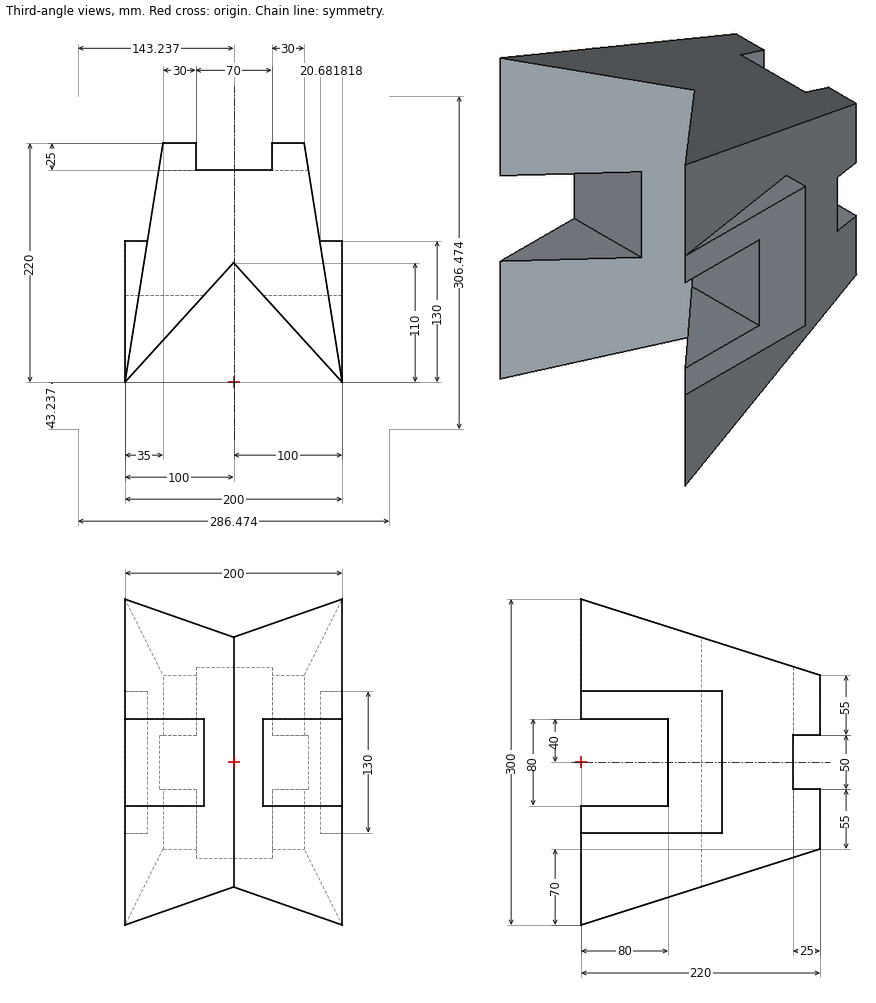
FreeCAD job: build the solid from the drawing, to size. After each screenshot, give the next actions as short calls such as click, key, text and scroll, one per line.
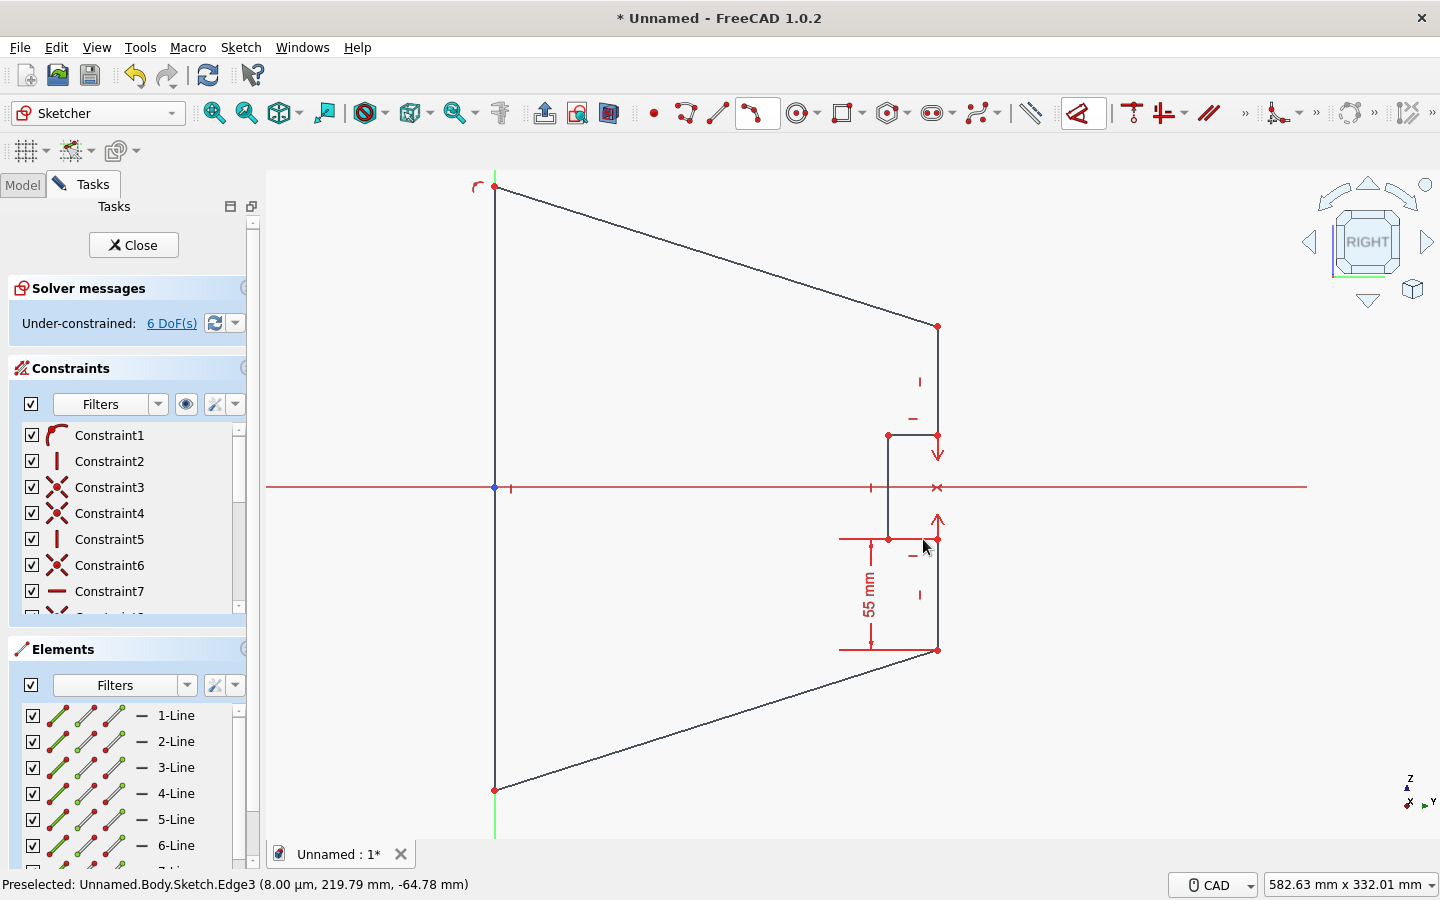
click(923, 539)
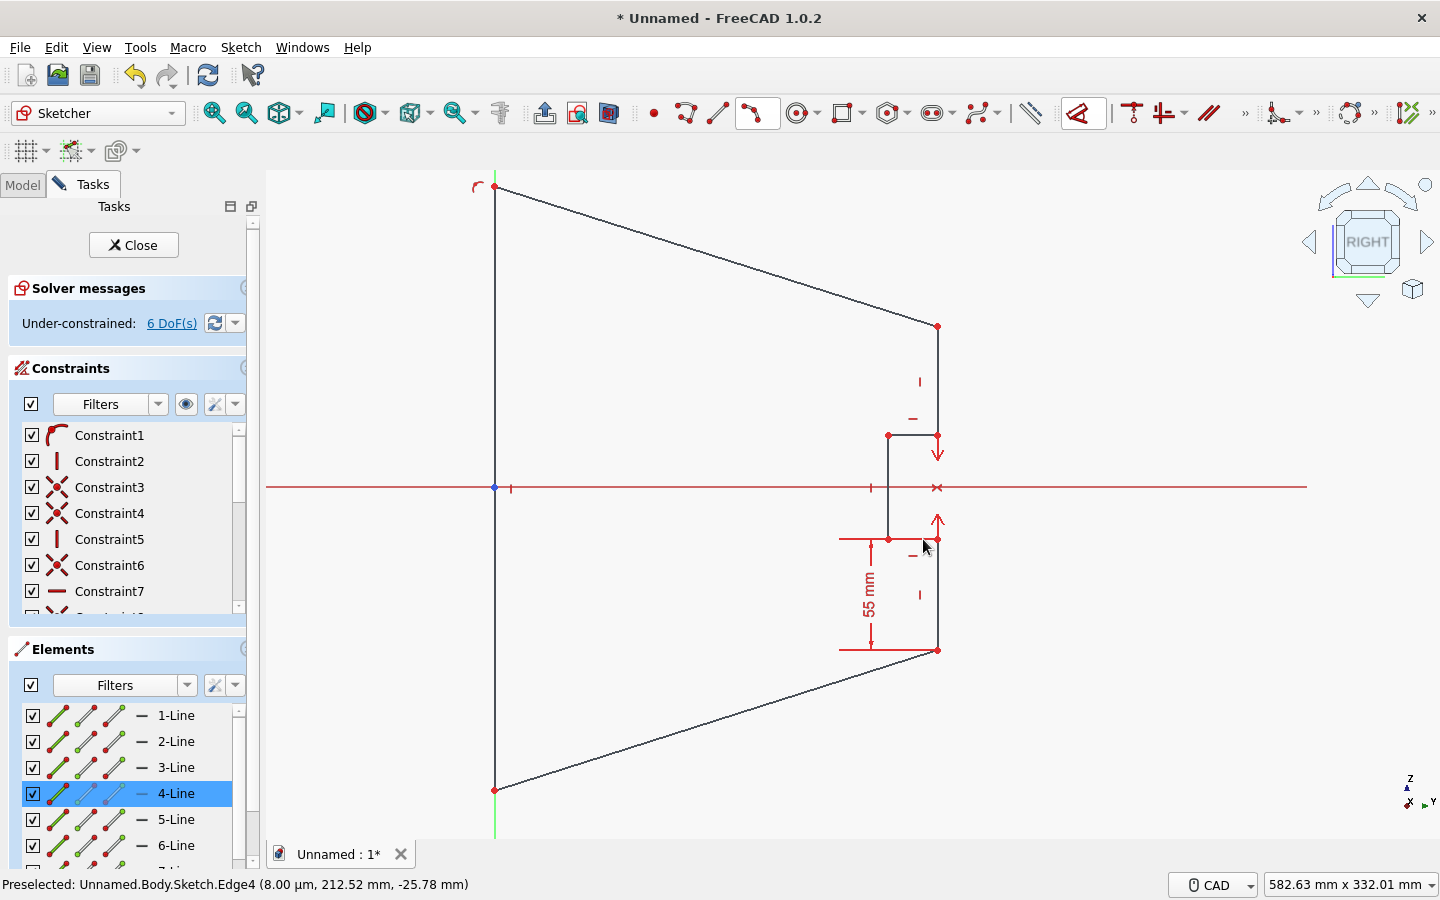
click(1100, 114)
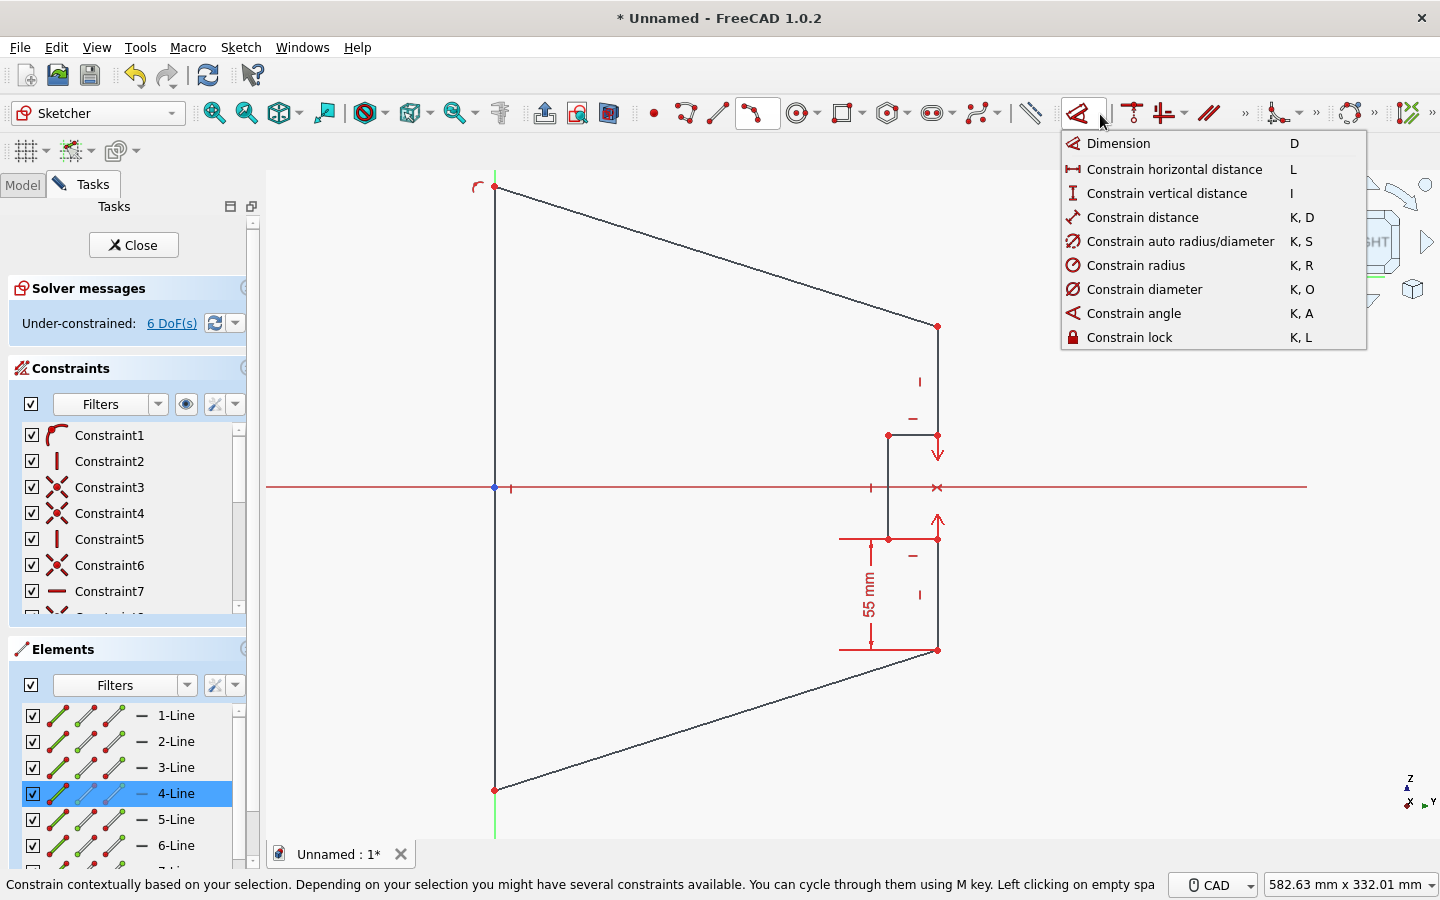
click(1214, 169)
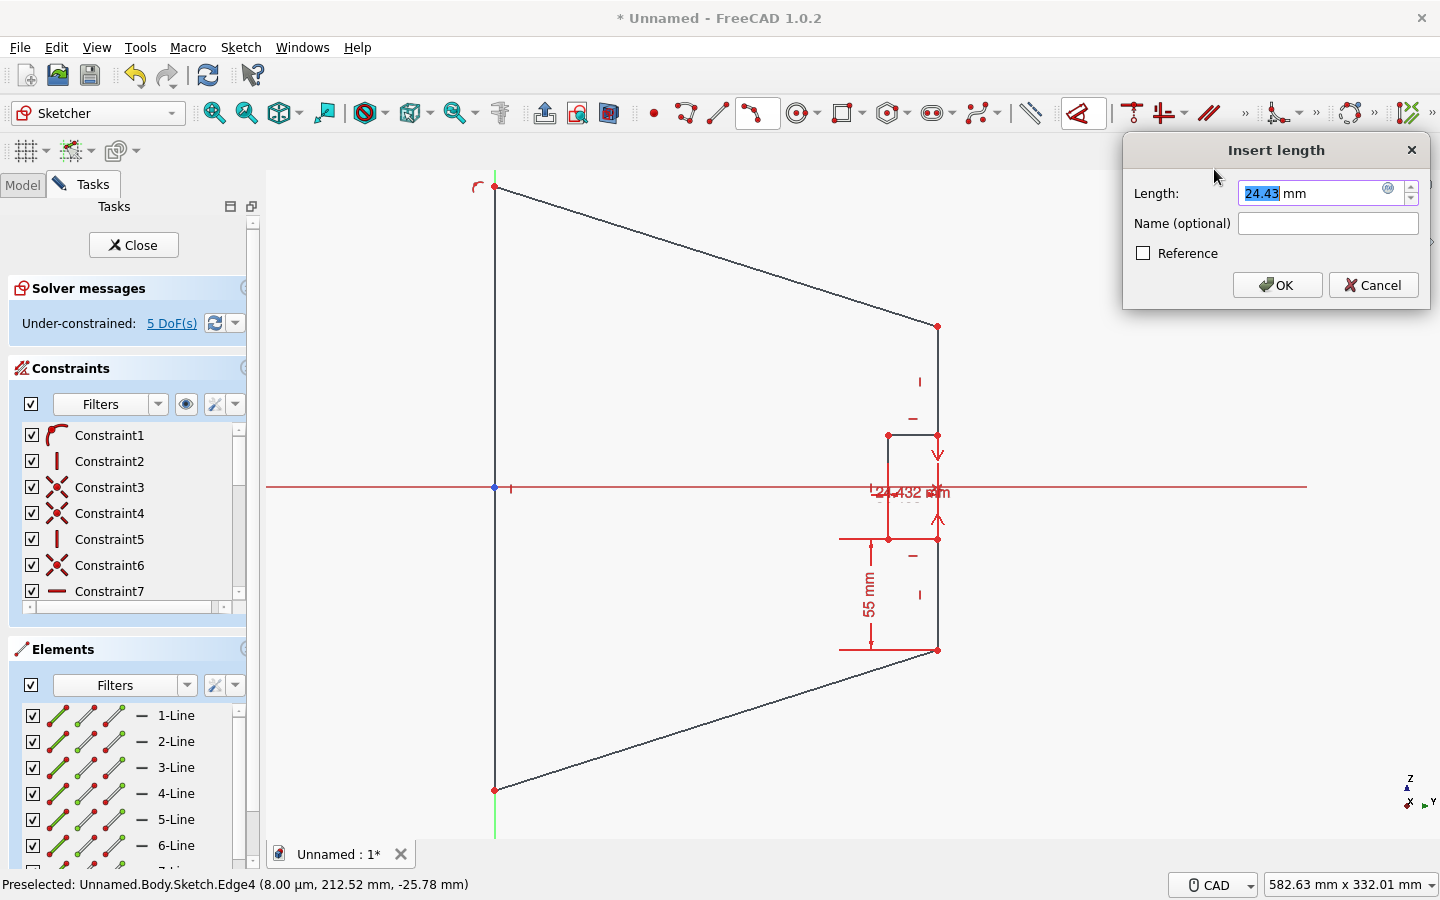
text(25)
key(Return)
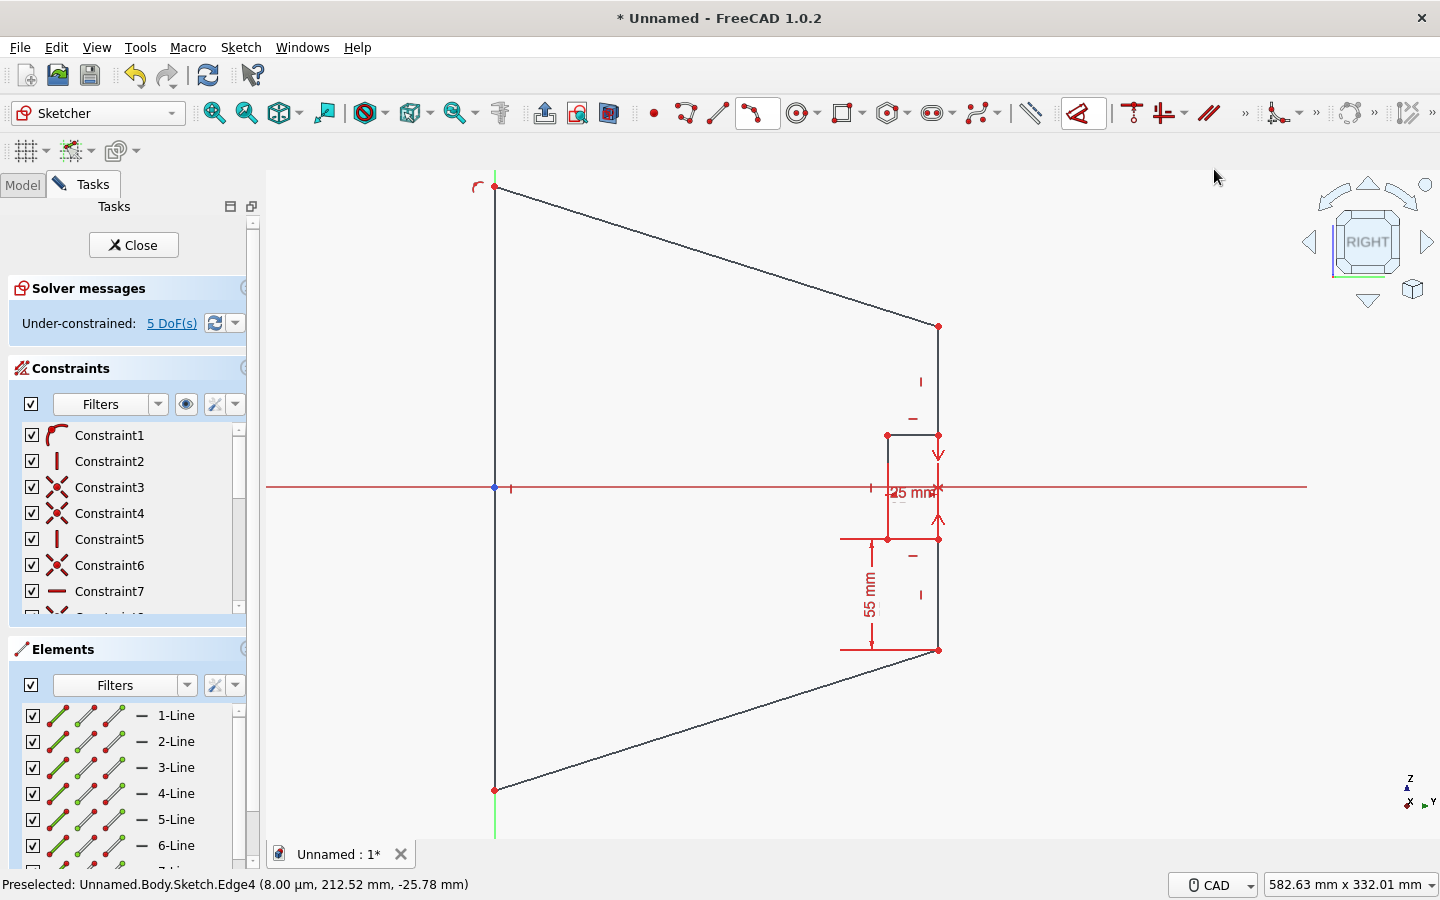
click(888, 508)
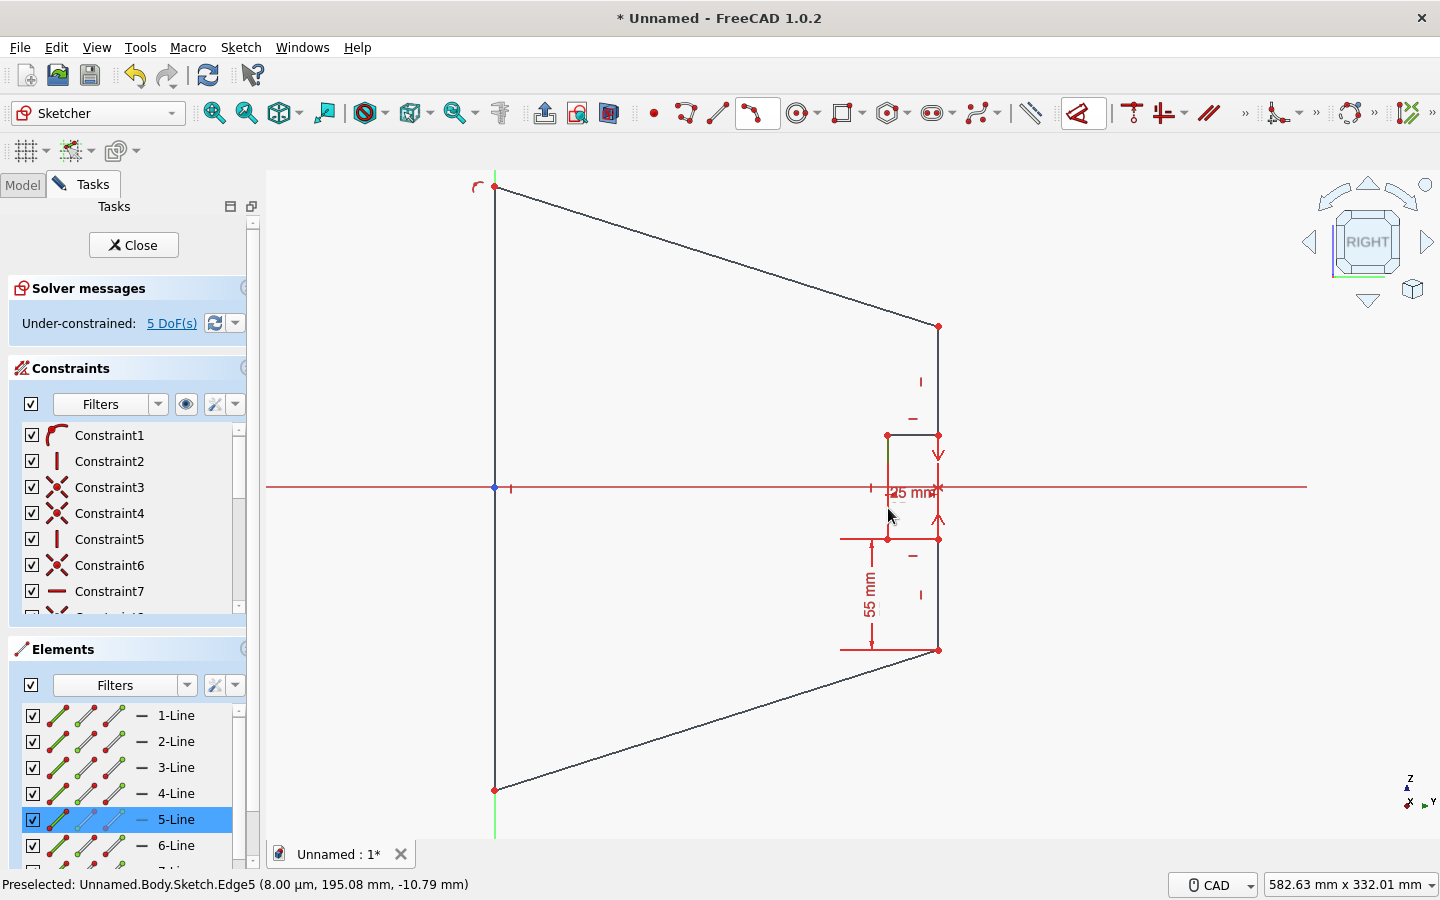
key(i)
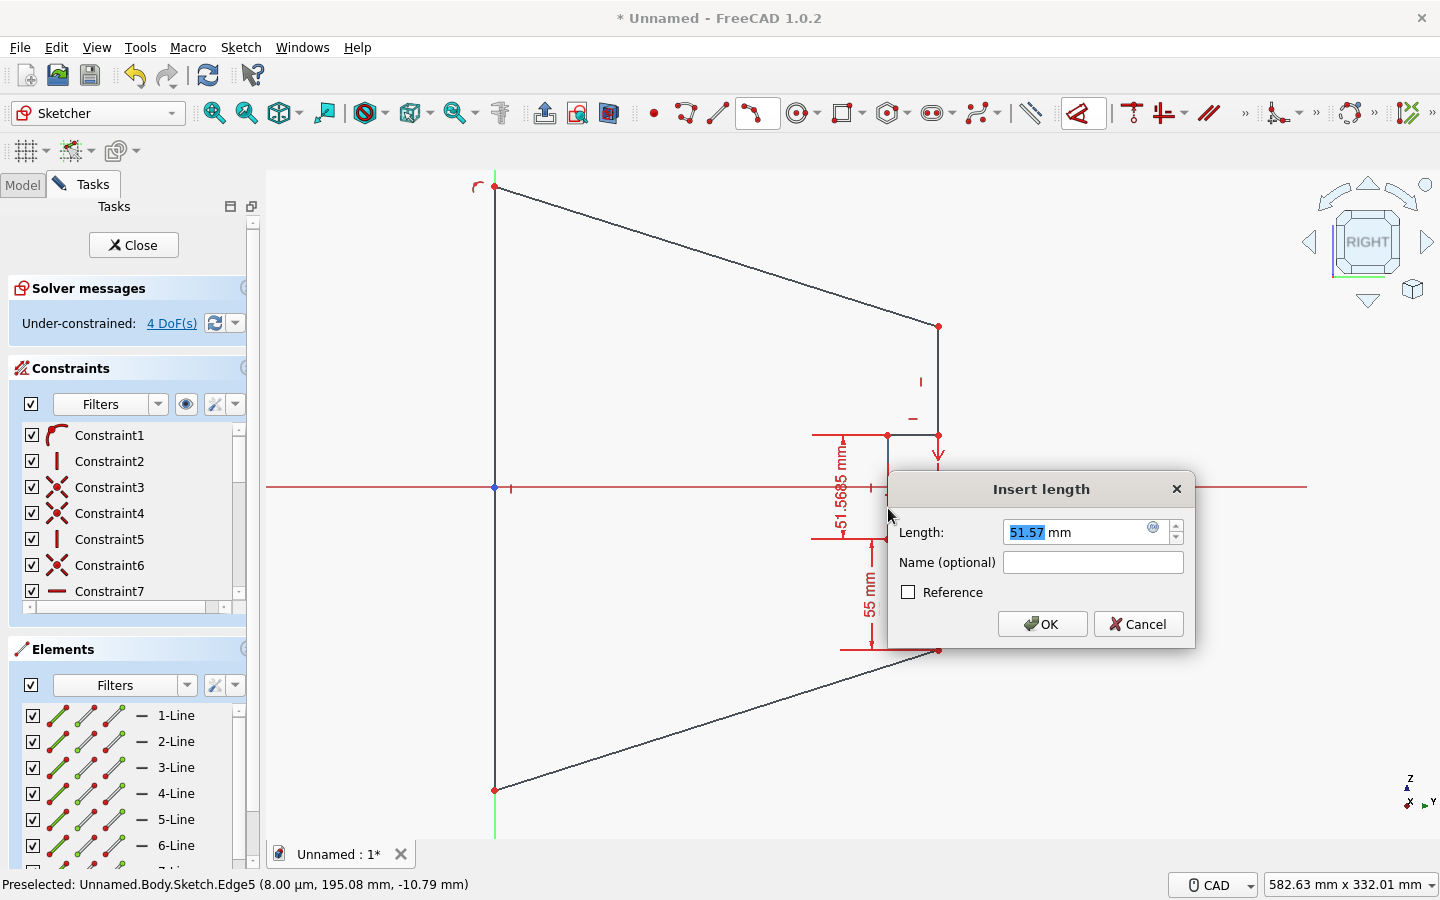
text(50)
key(Return)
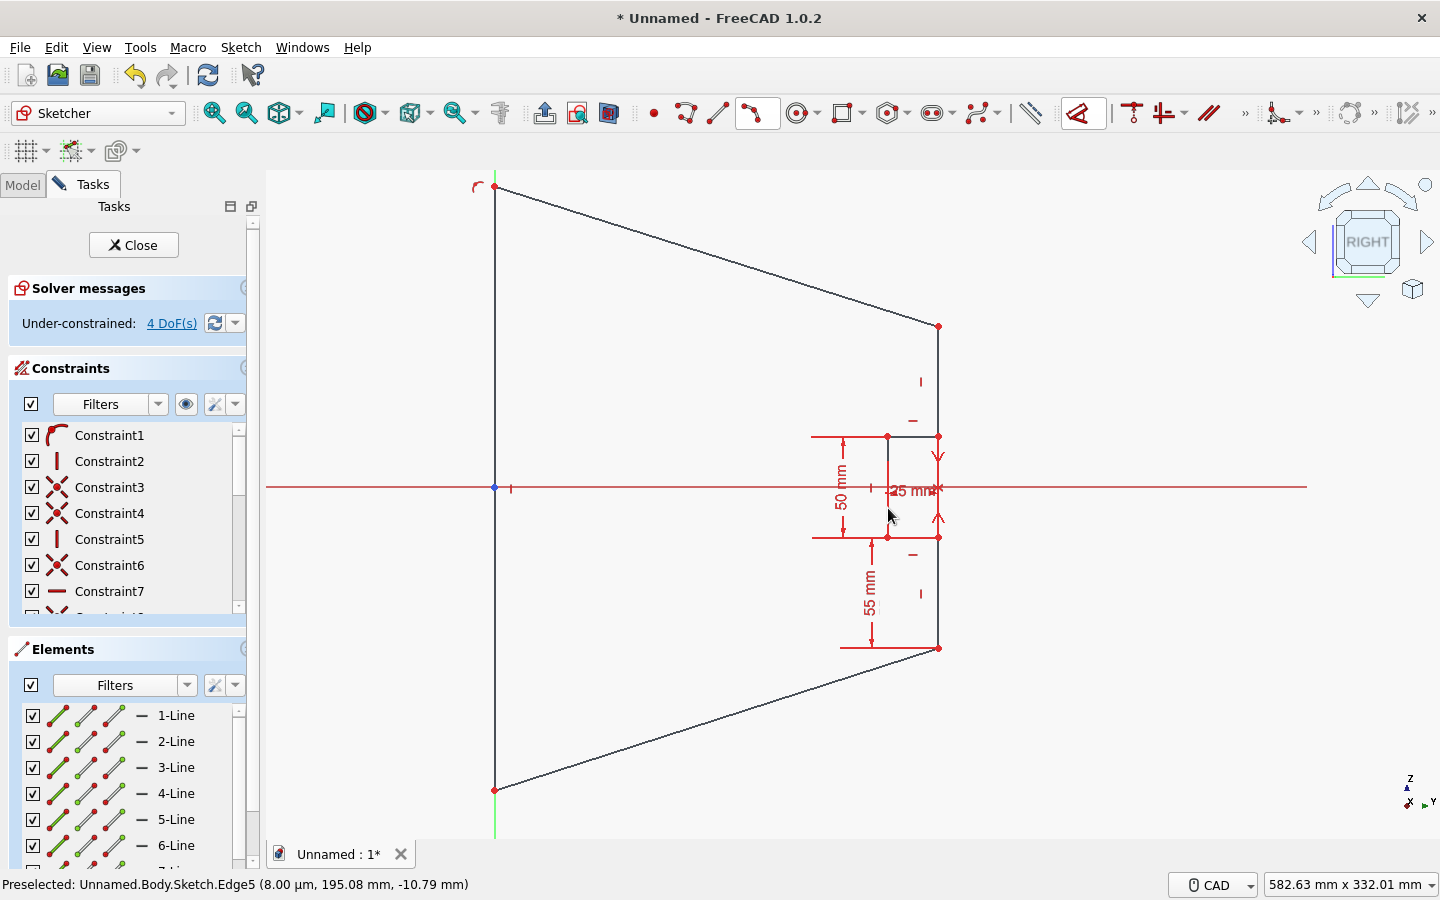
click(938, 404)